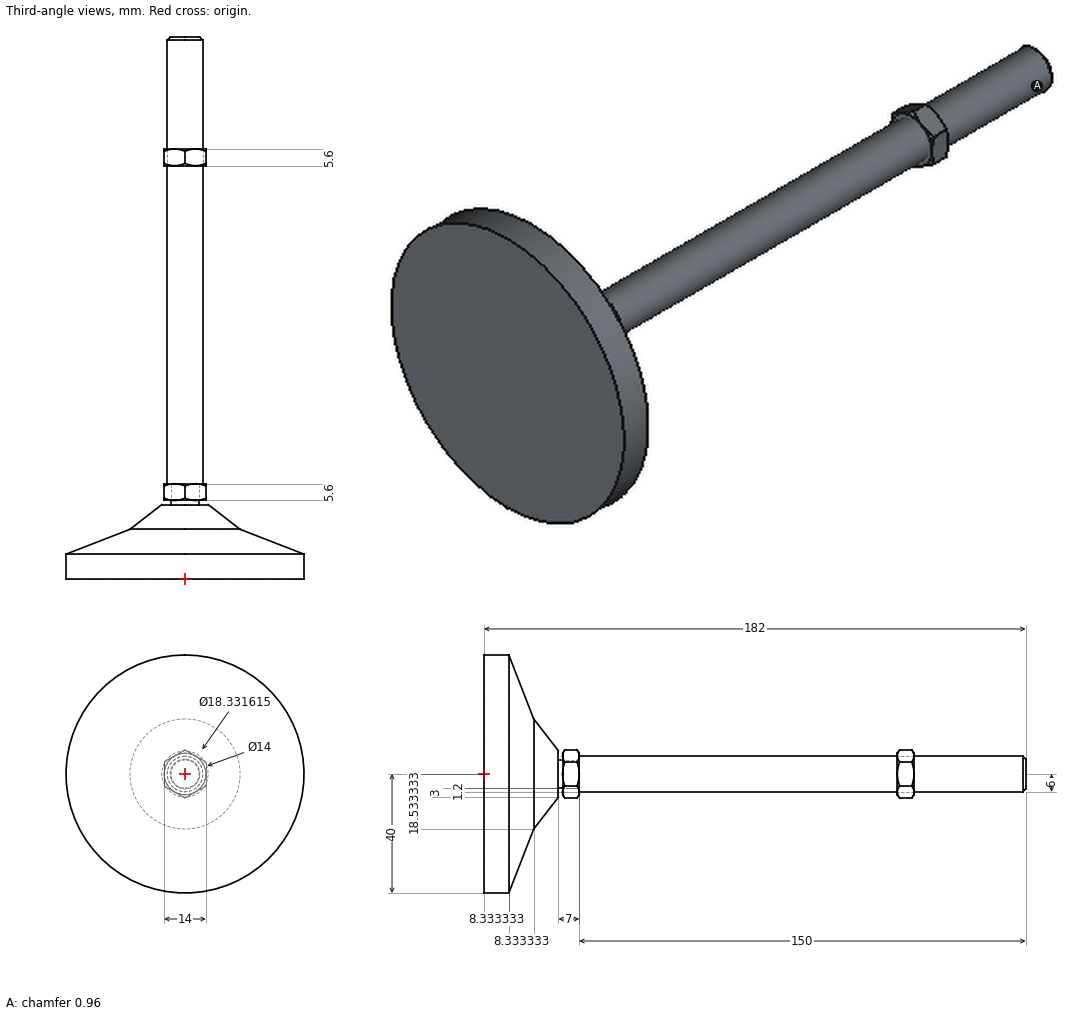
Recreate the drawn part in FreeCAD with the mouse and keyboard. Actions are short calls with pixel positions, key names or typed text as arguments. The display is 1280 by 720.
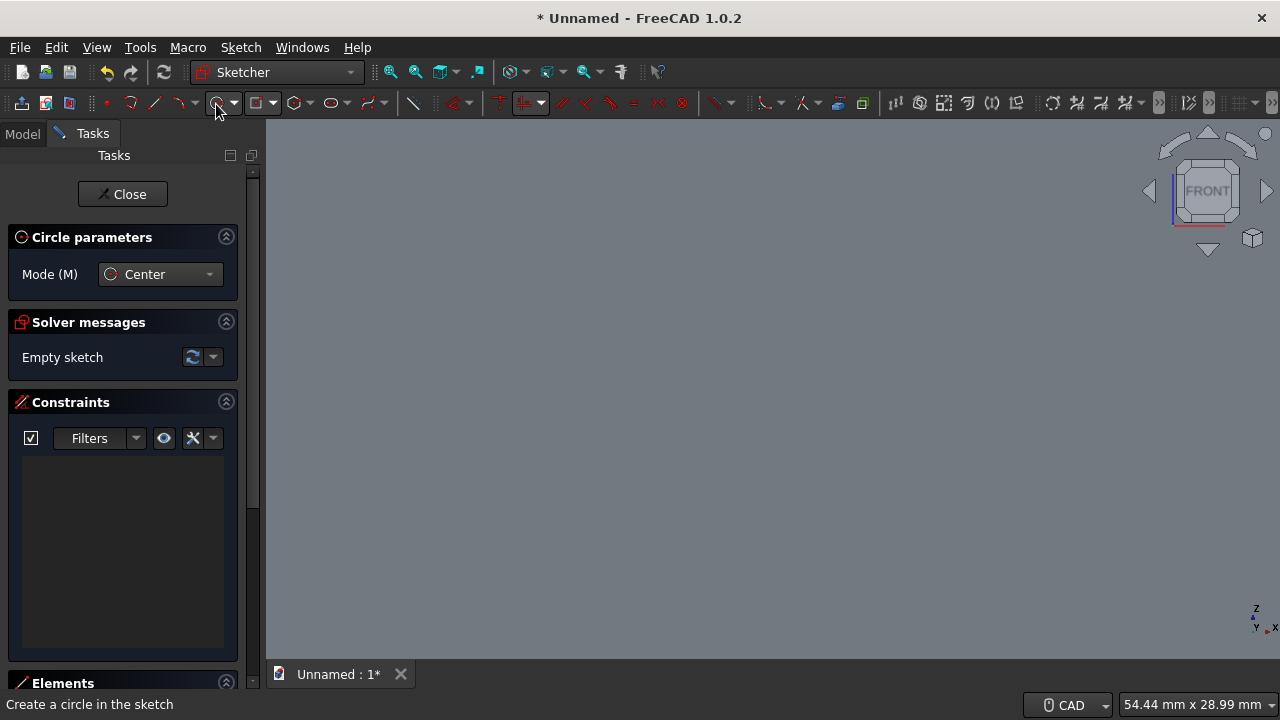
click(699, 386)
click(820, 265)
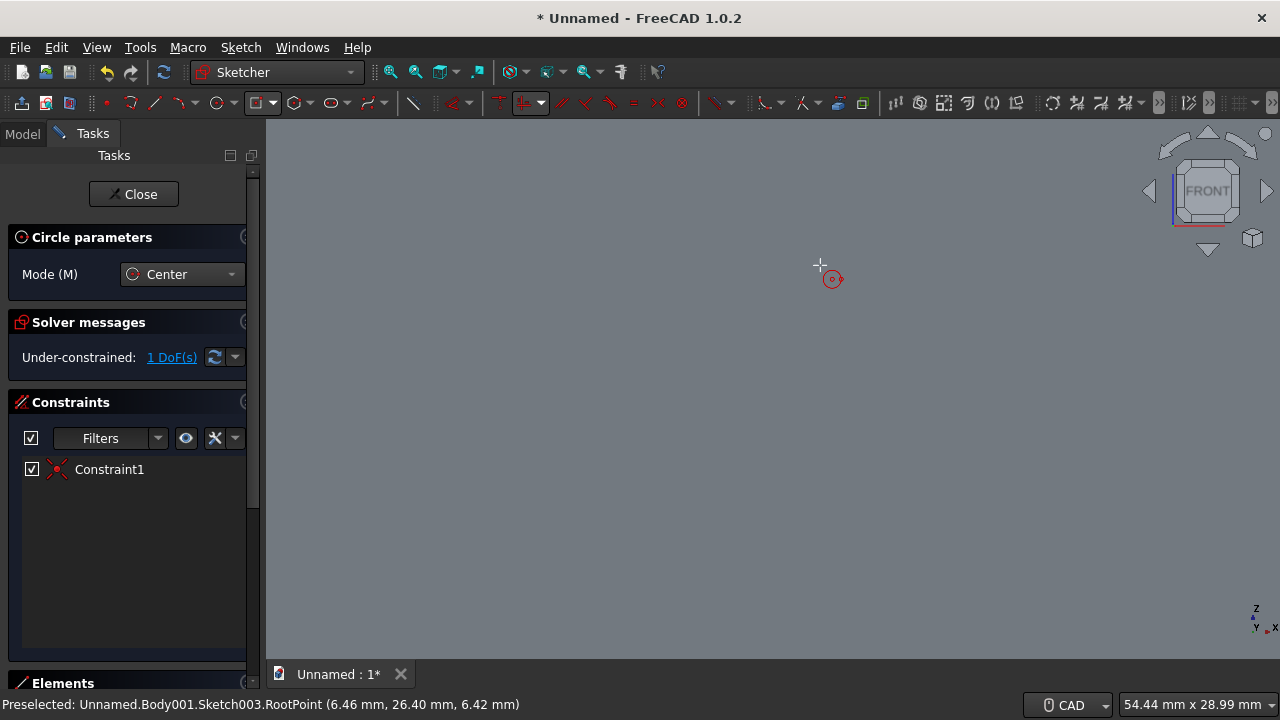
click(699, 386)
click(792, 294)
key(Escape)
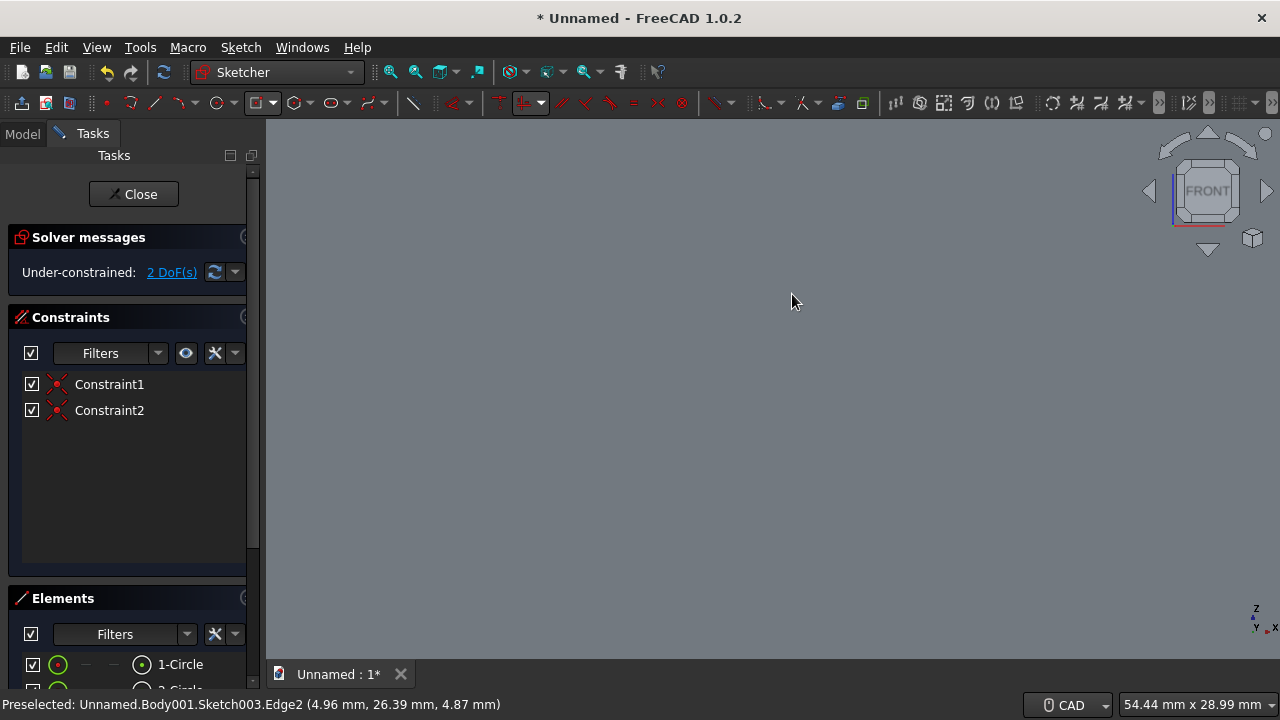
key(d)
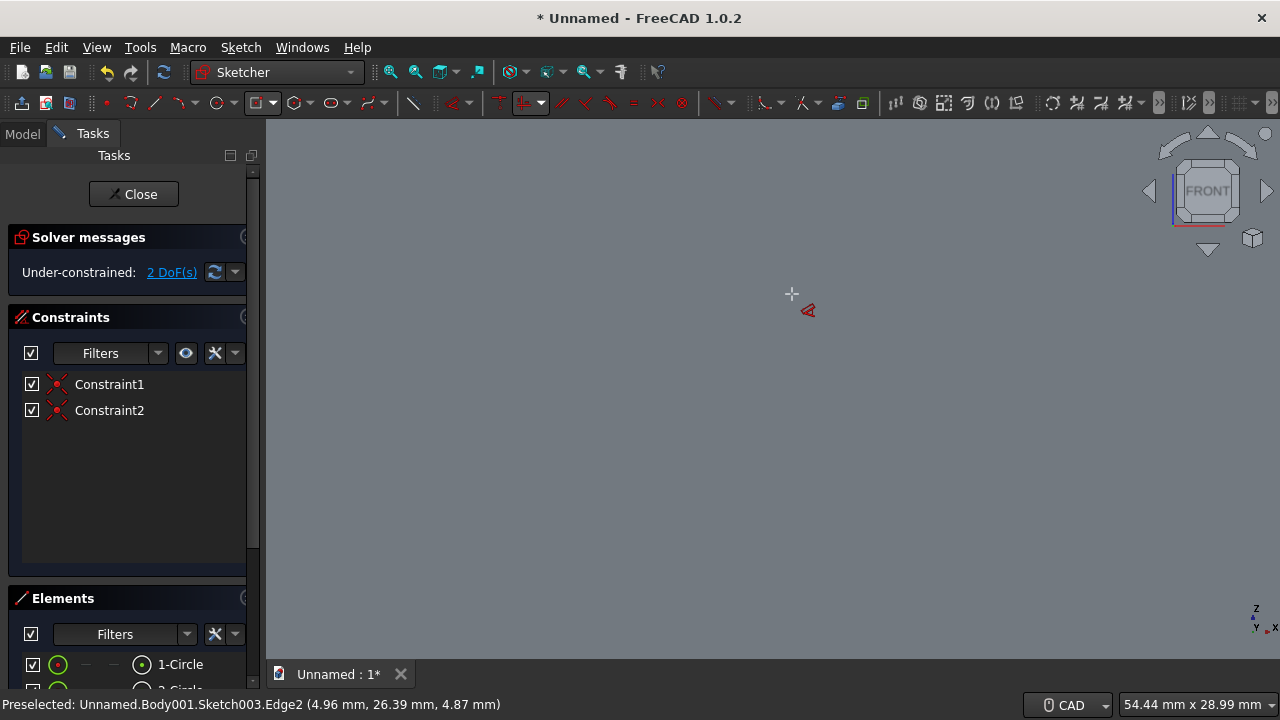
click(819, 265)
click(842, 242)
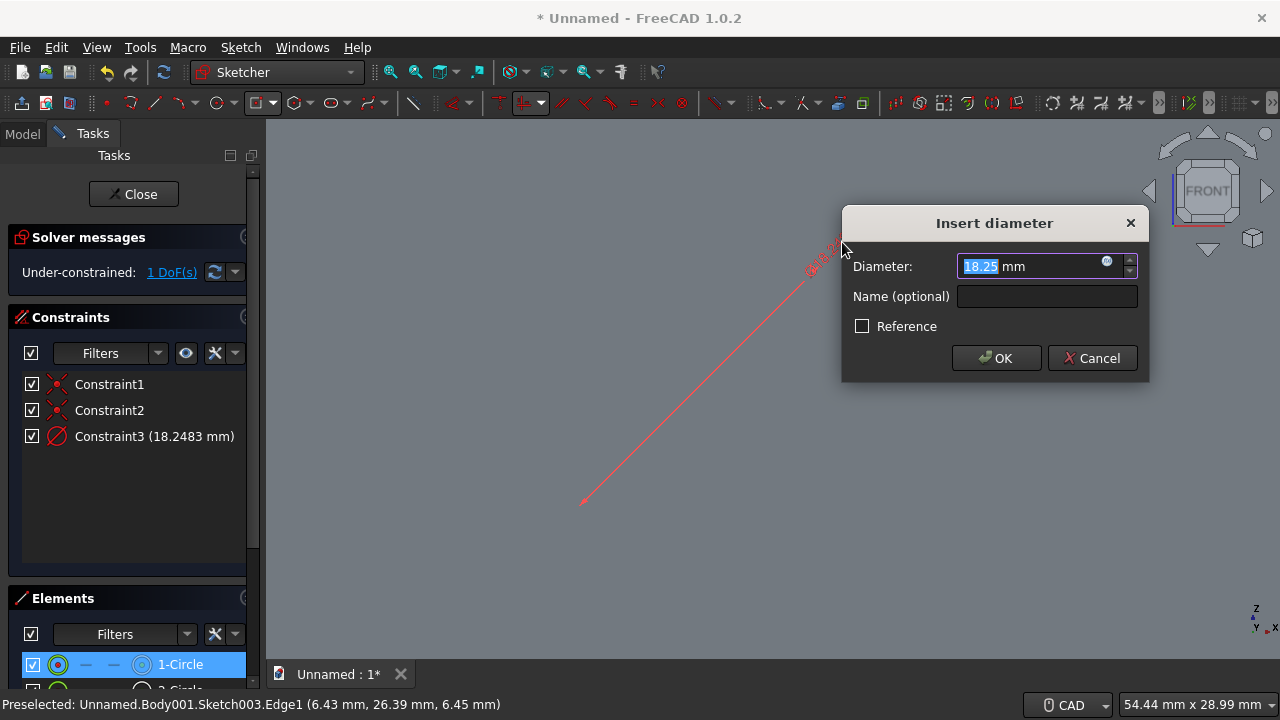
text(18.331615)
key(Return)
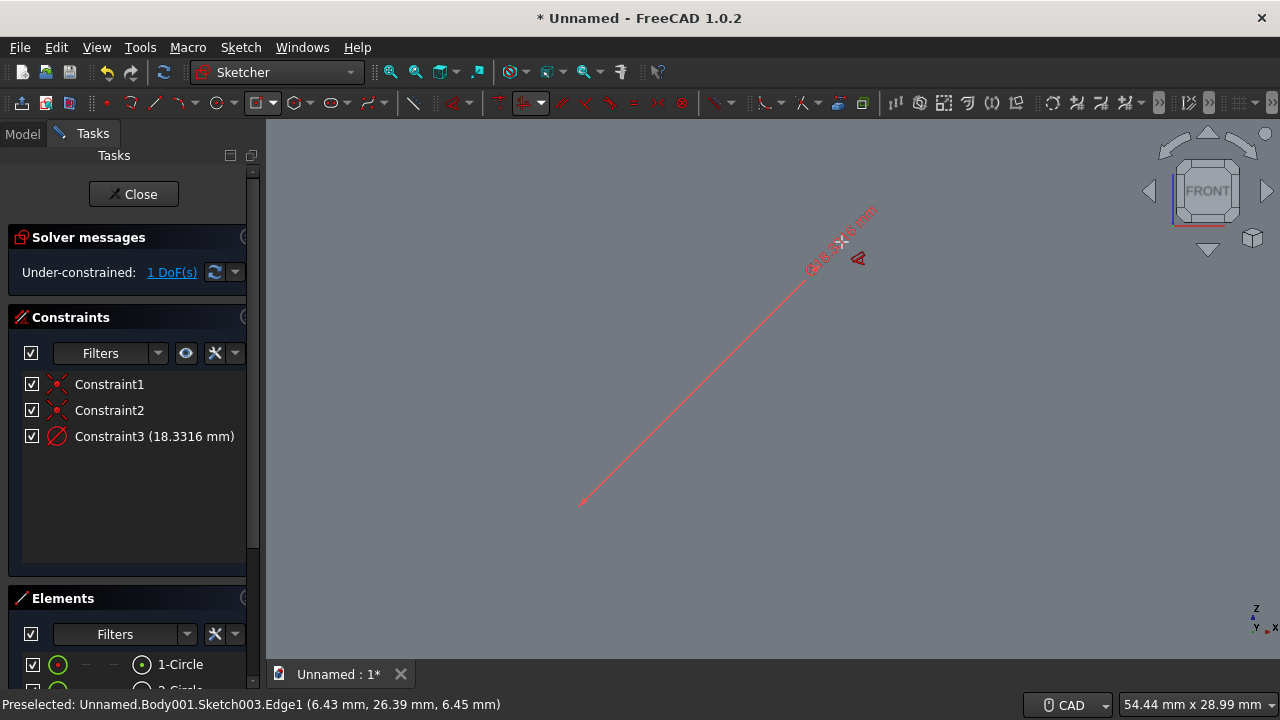
click(791, 294)
click(877, 334)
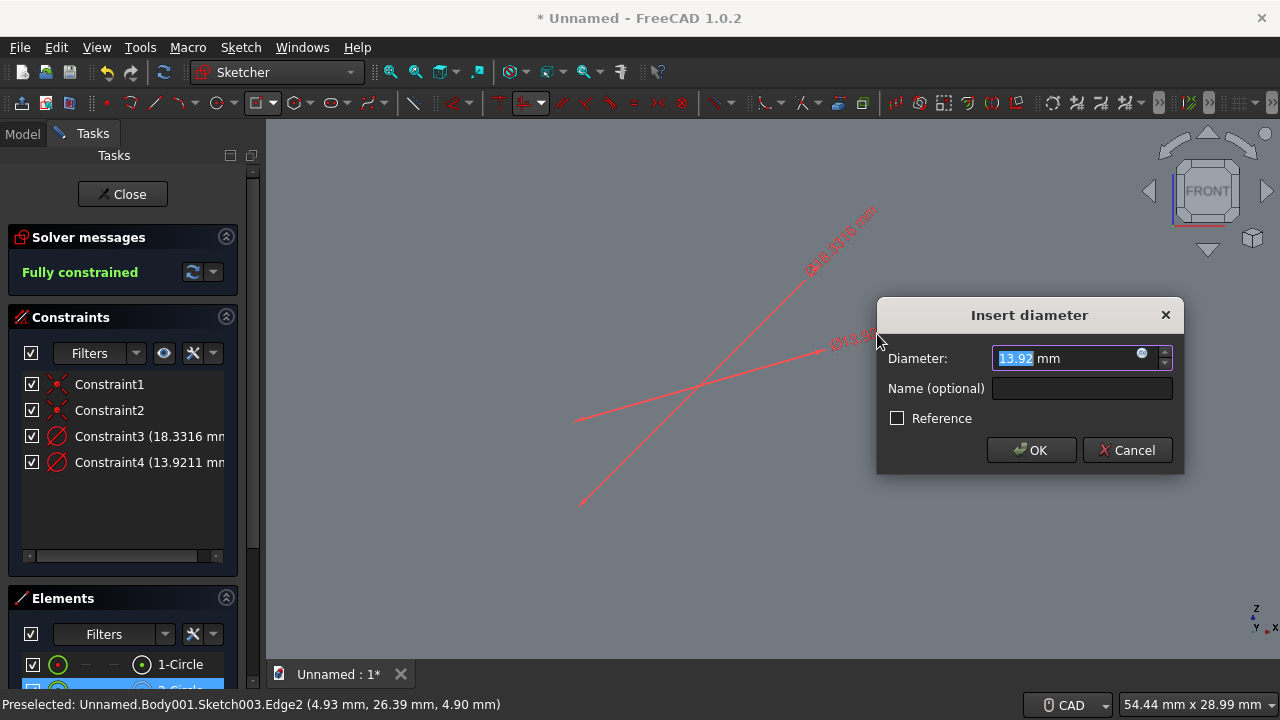
text(14)
key(Return)
key(Escape)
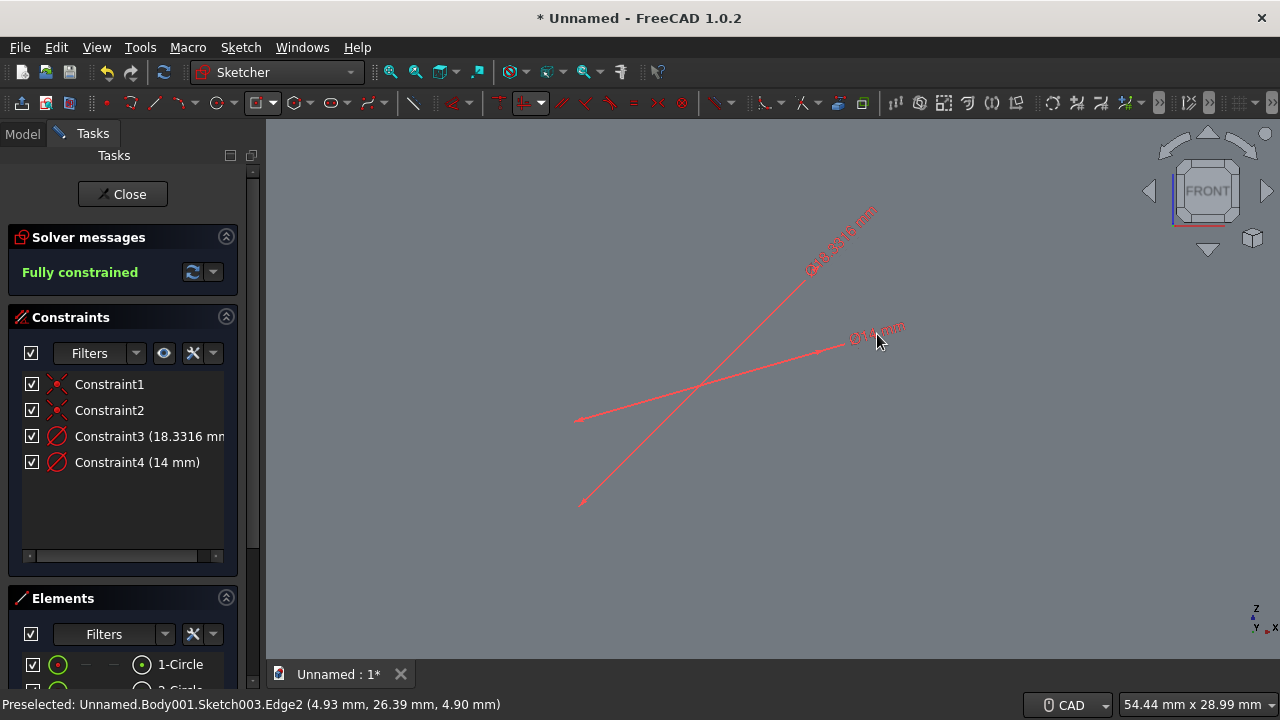
click(123, 194)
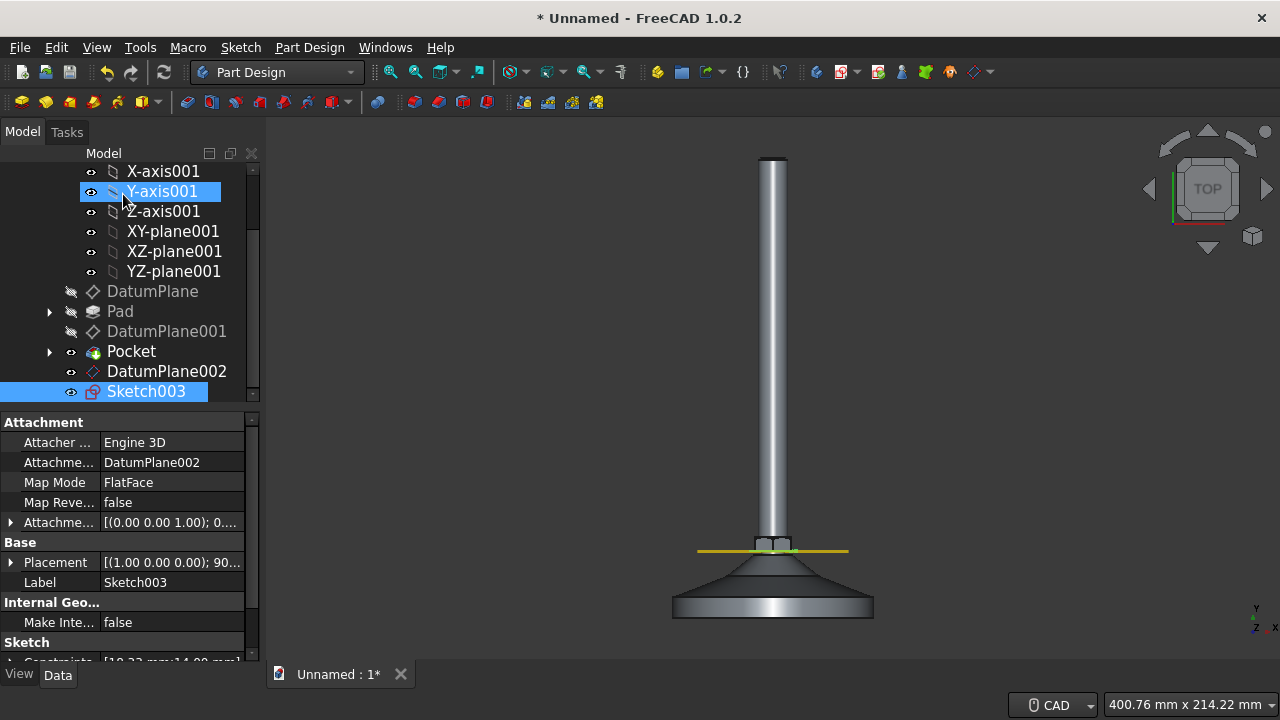
click(188, 102)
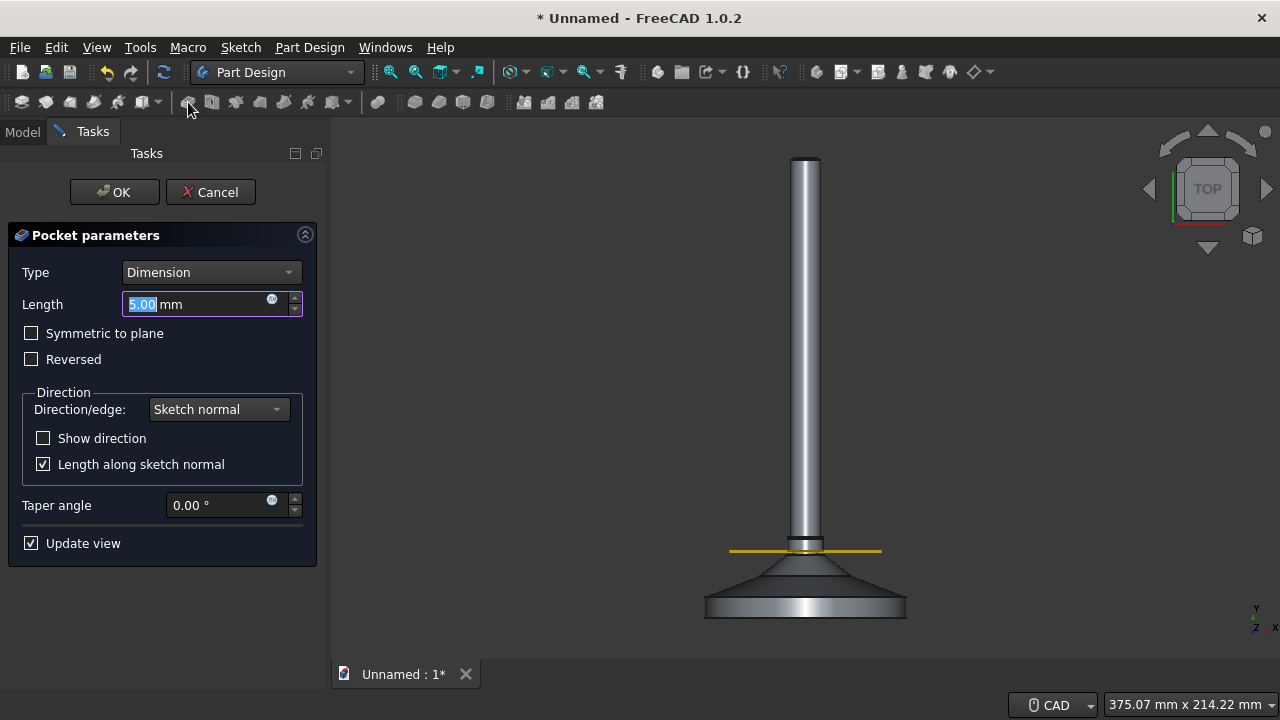
text(5.6)
key(Tab)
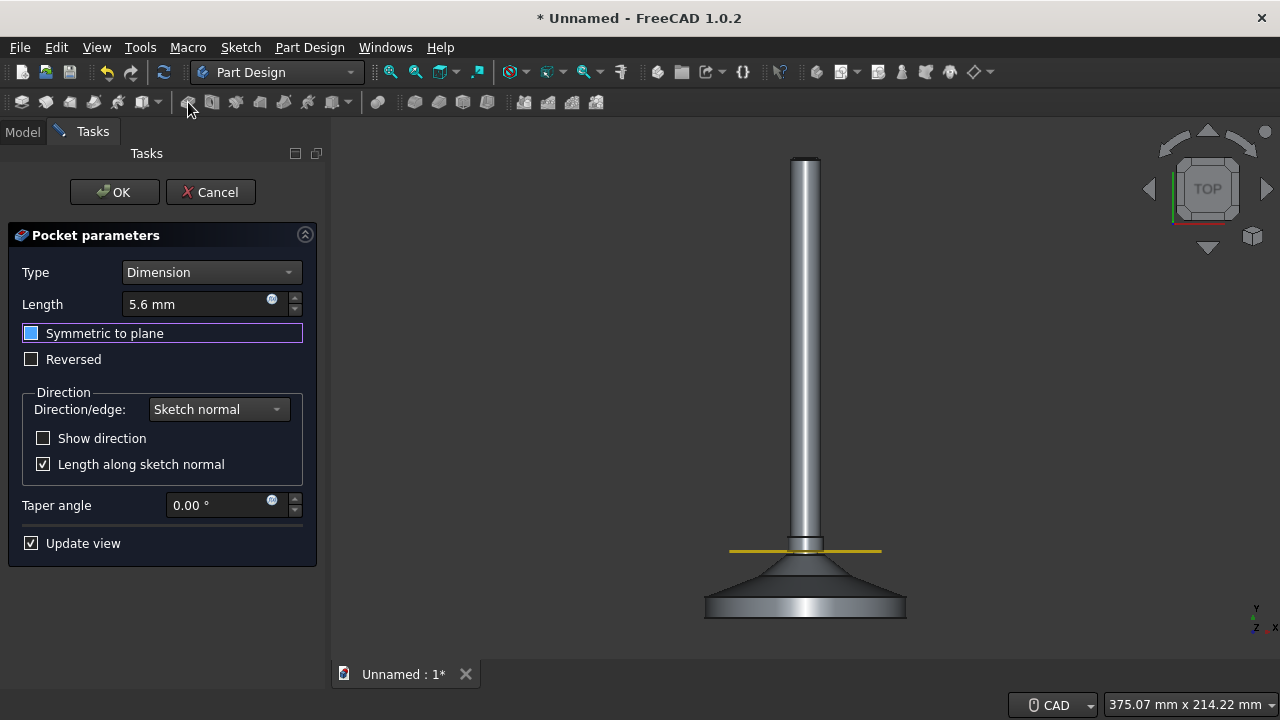
triple_click(226, 505)